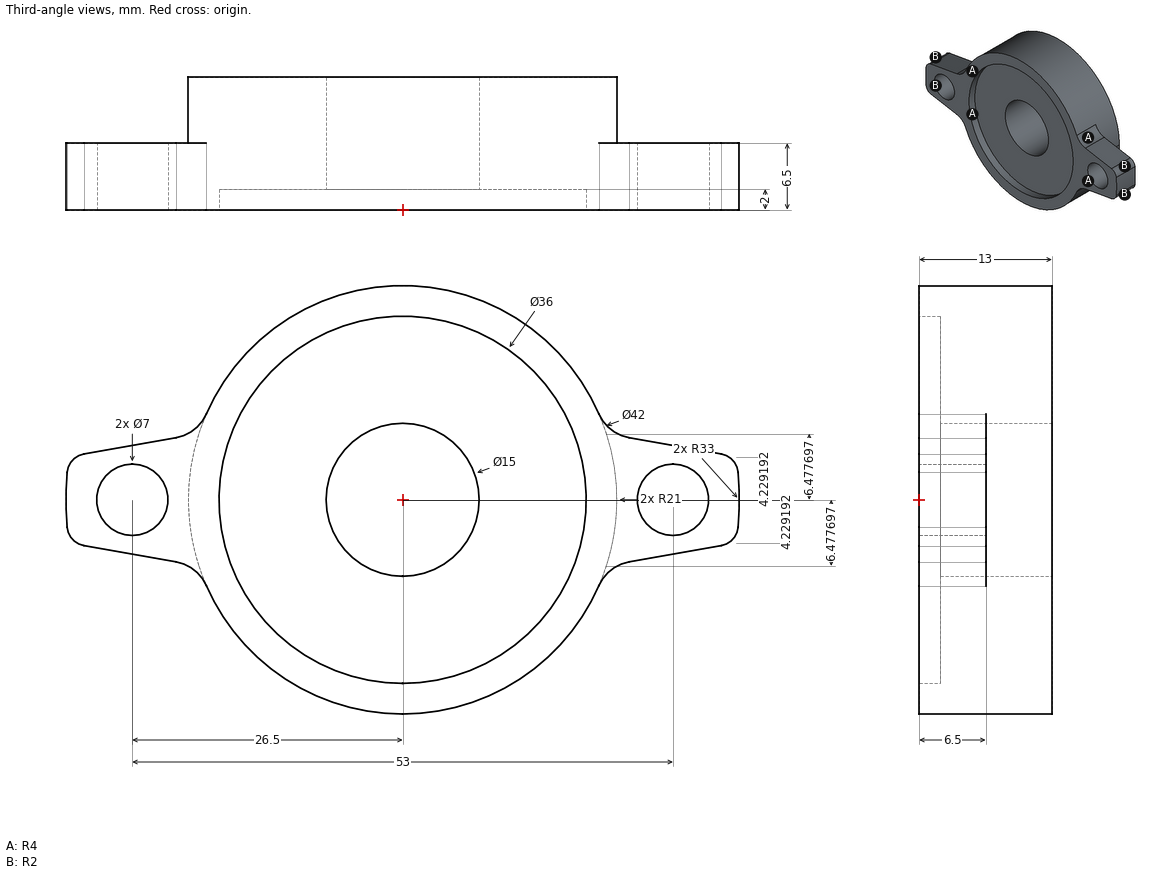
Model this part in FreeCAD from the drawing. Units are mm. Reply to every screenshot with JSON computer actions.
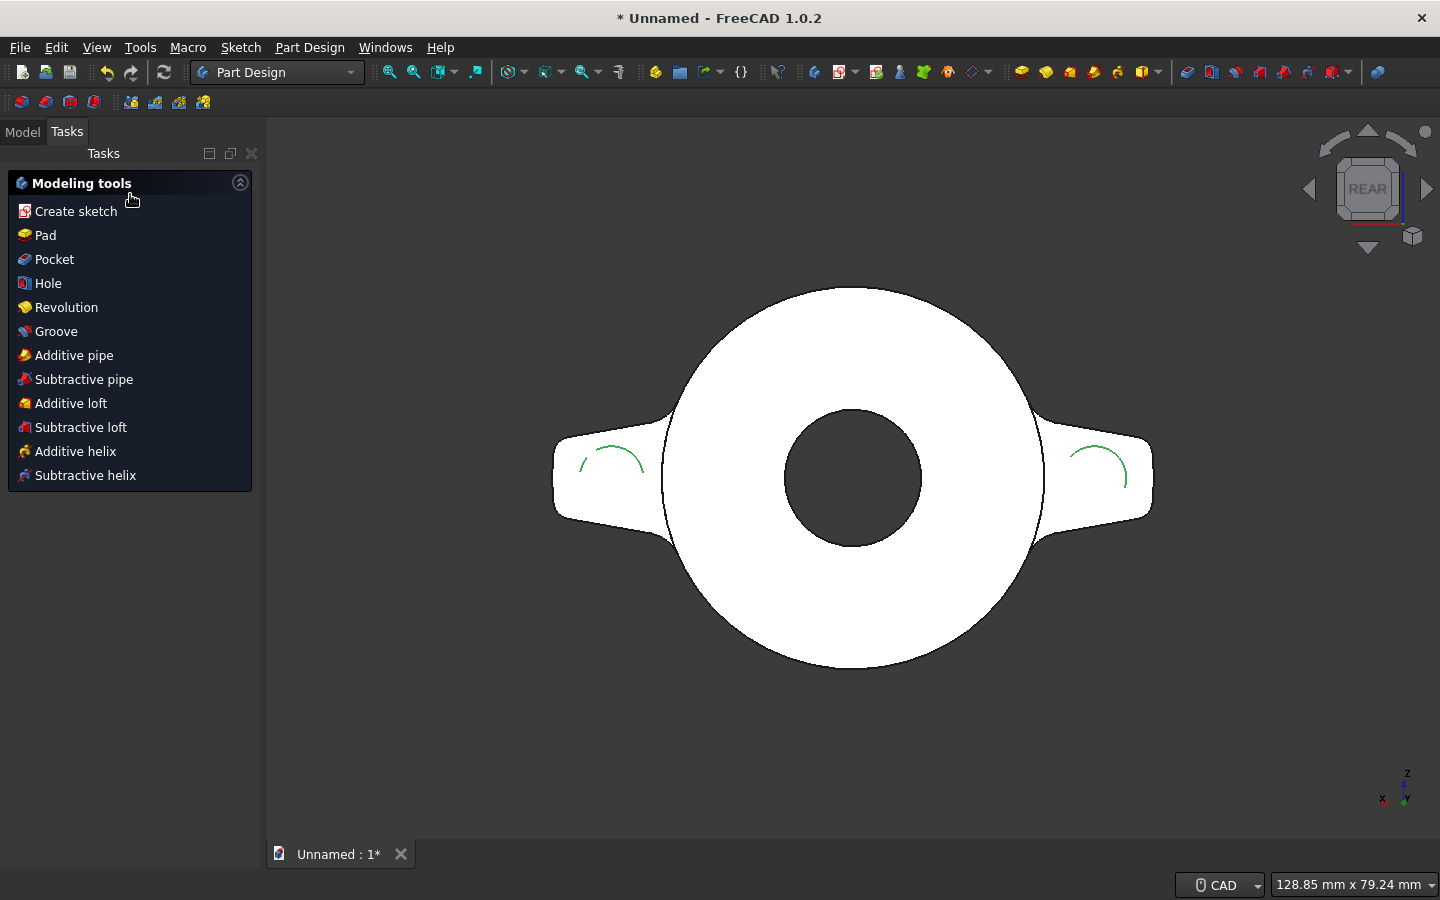
{"action": "left_click", "coordinate": [1188, 72]}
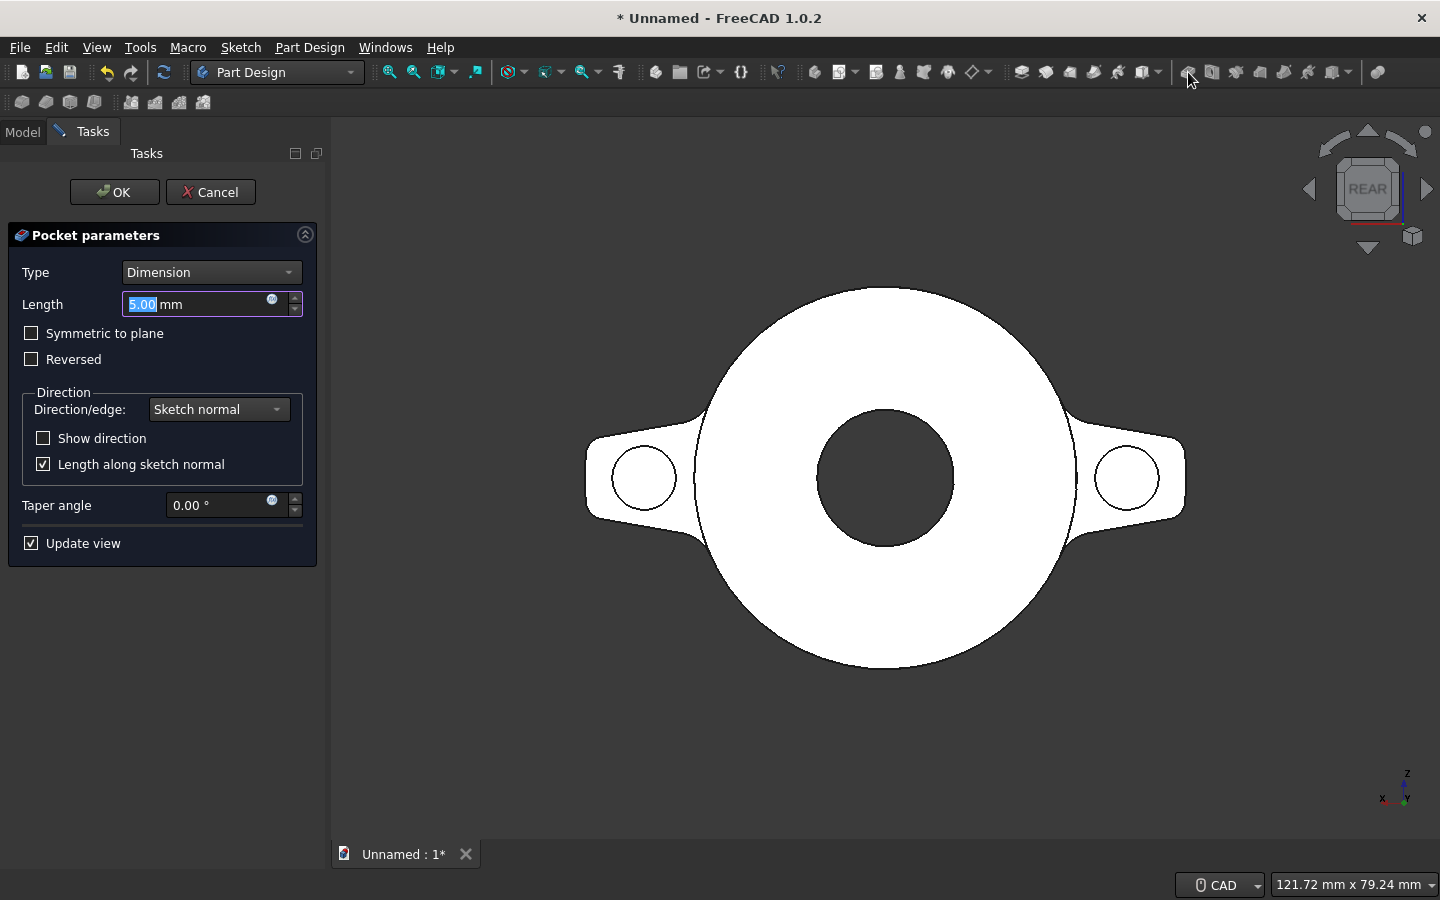
{"action": "type", "text": "6.5"}
{"action": "key", "text": "Tab"}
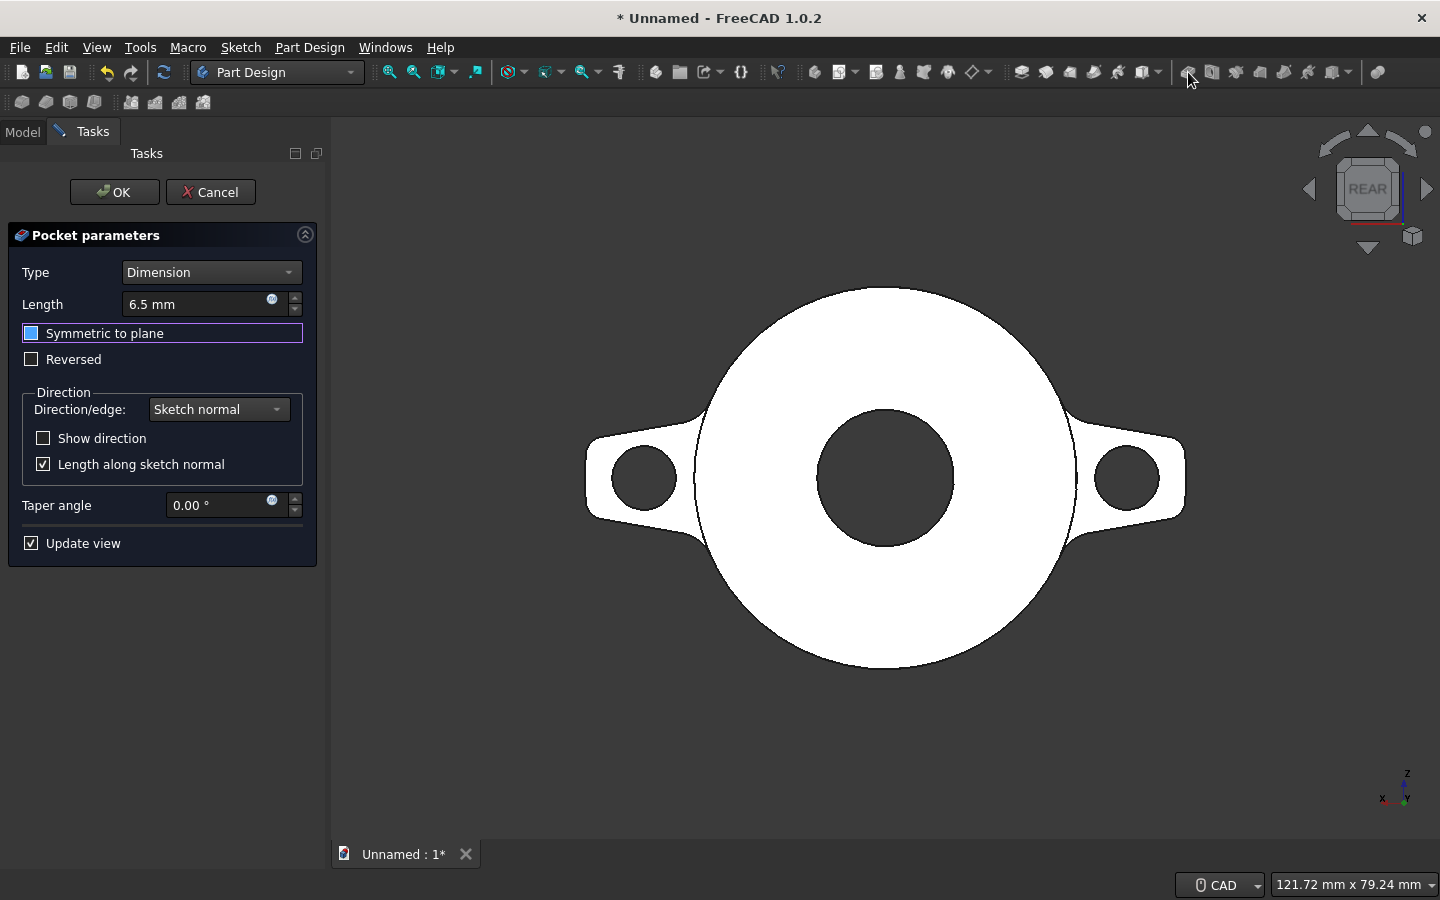
{"action": "left_click", "coordinate": [115, 192]}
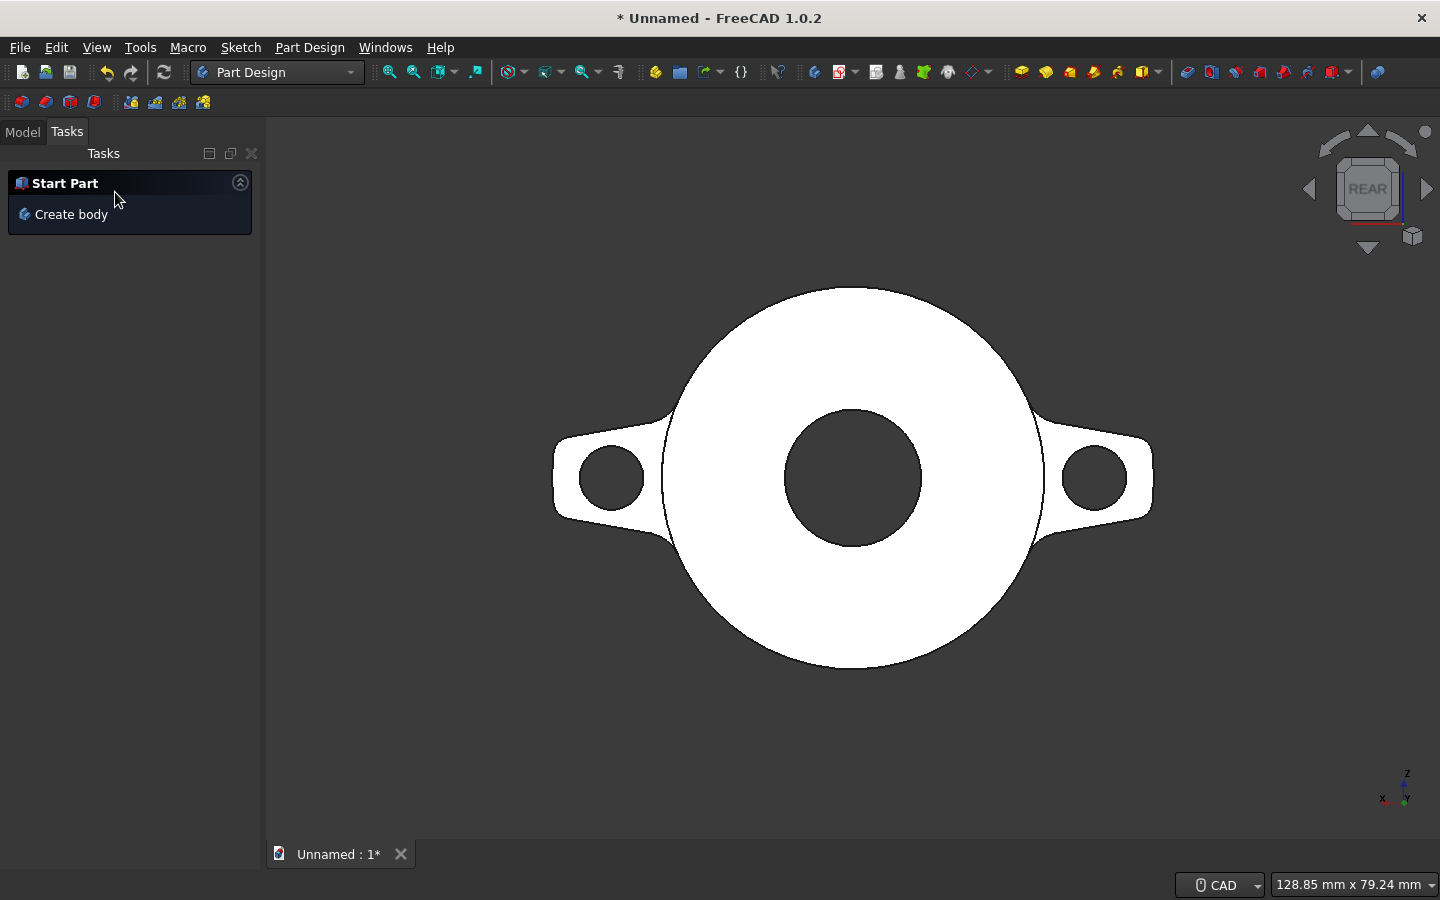
{"action": "left_click", "coordinate": [840, 72]}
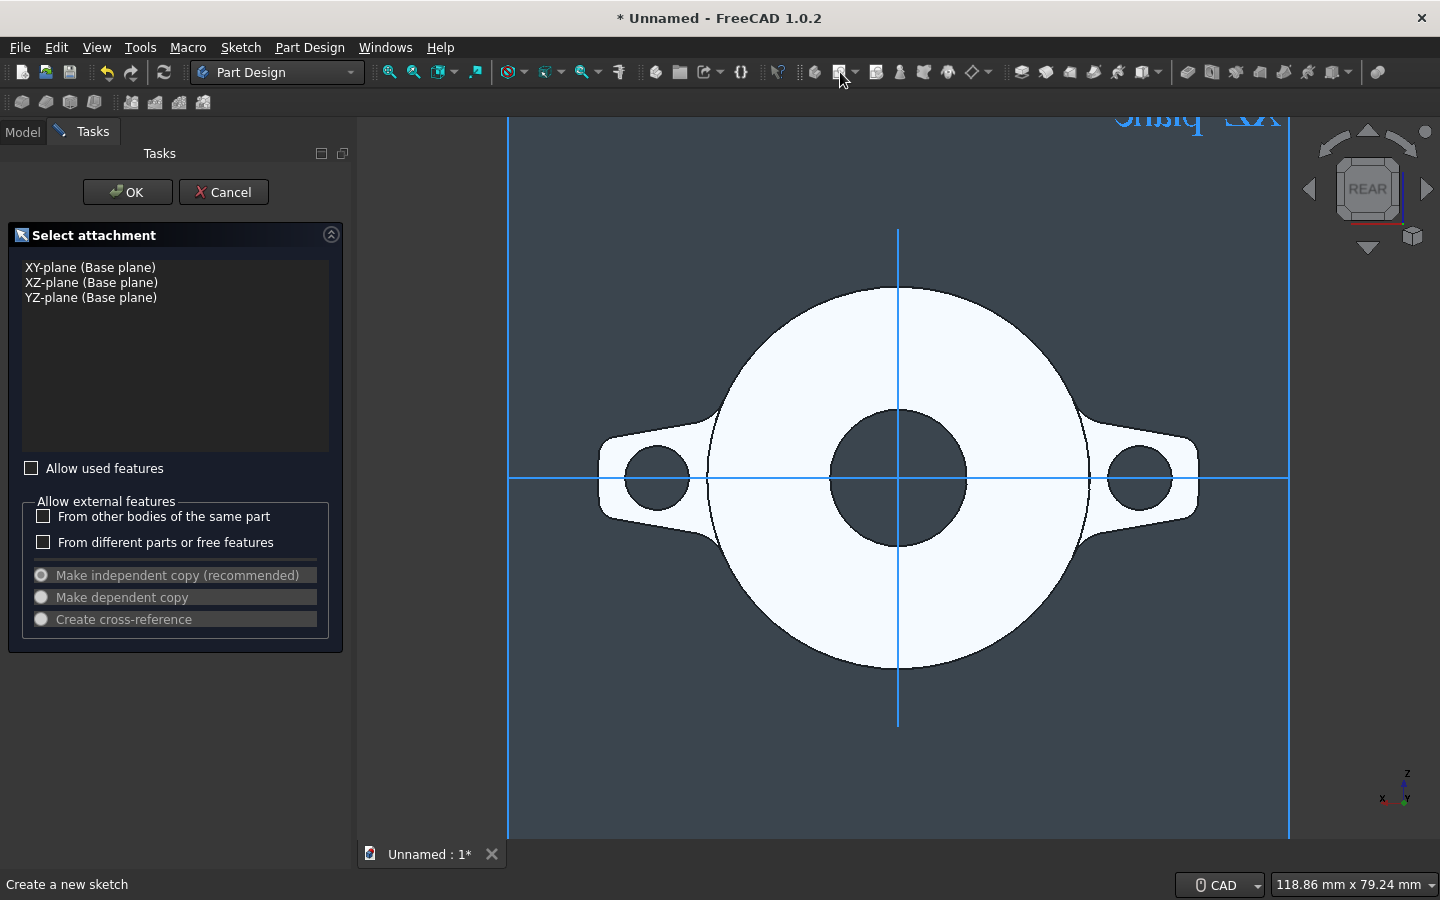
{"action": "left_click", "coordinate": [82, 282]}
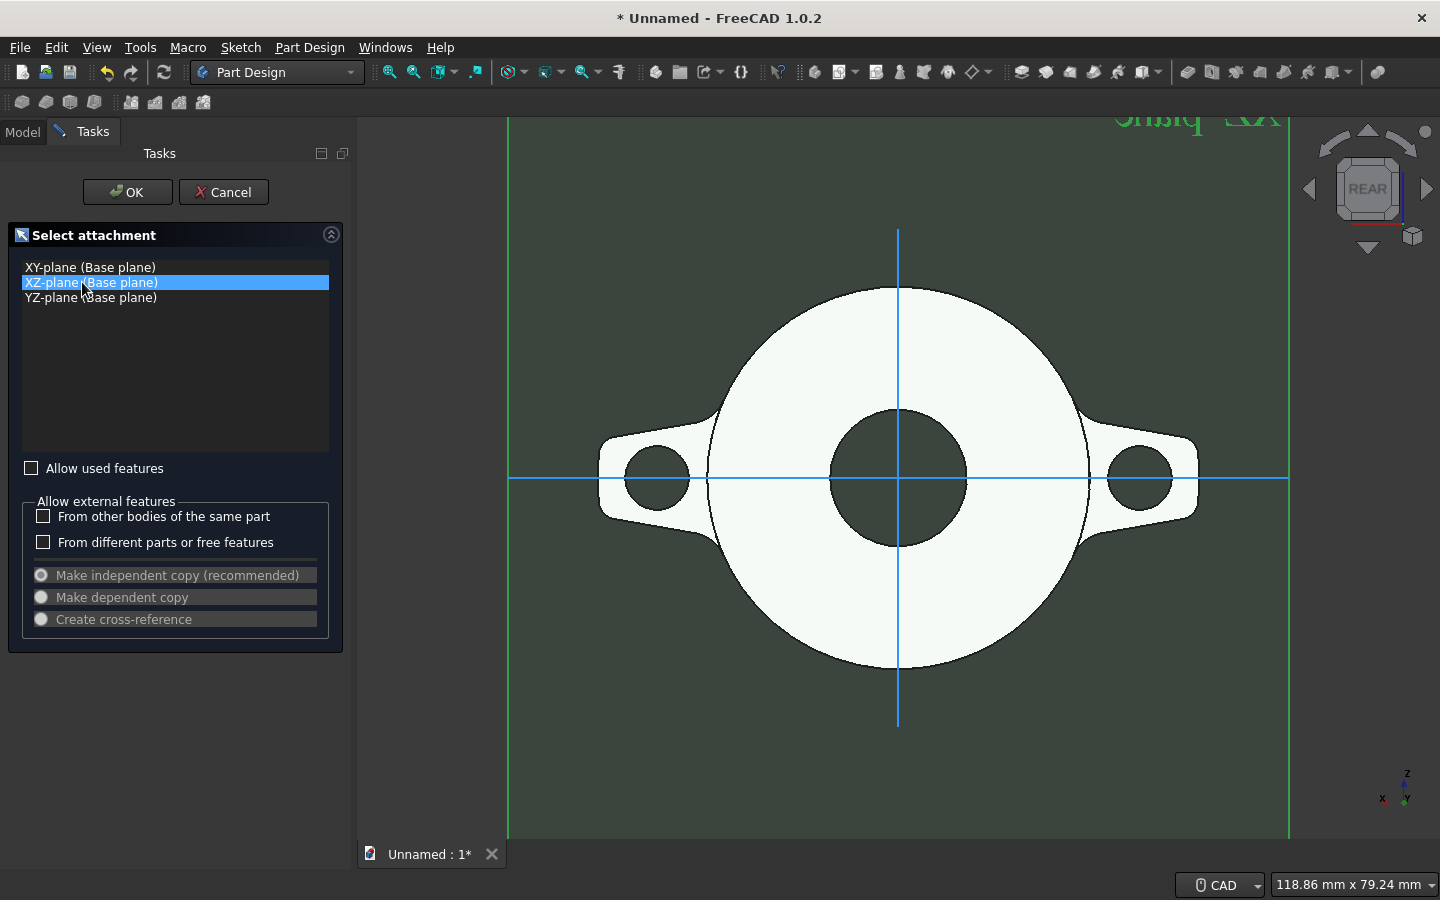
{"action": "left_click", "coordinate": [128, 192]}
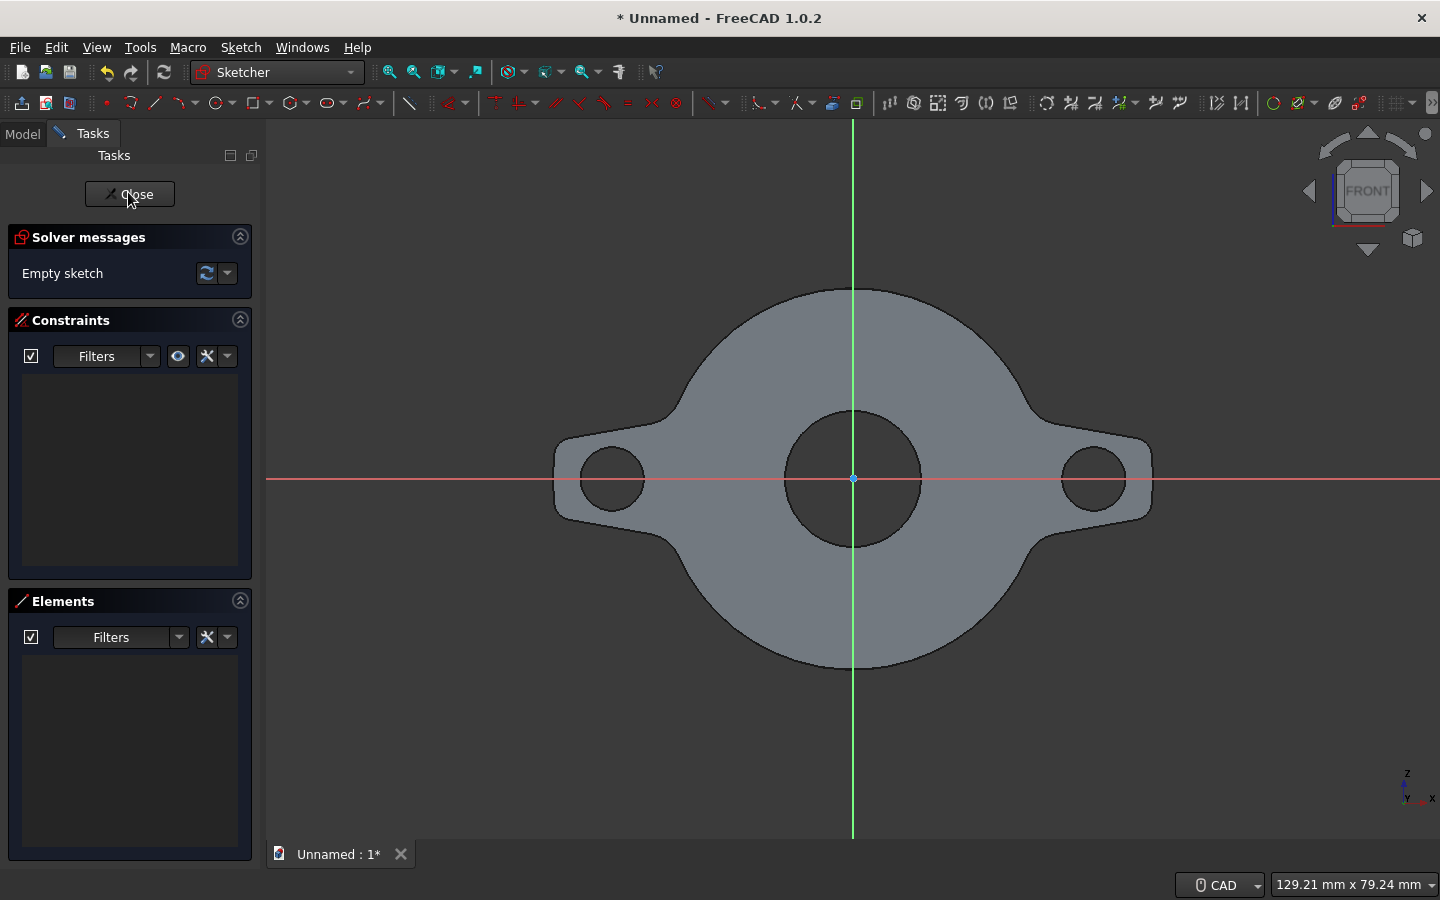
{"action": "scroll", "coordinate": [992, 479], "scroll_direction": "up", "scroll_amount": 2}